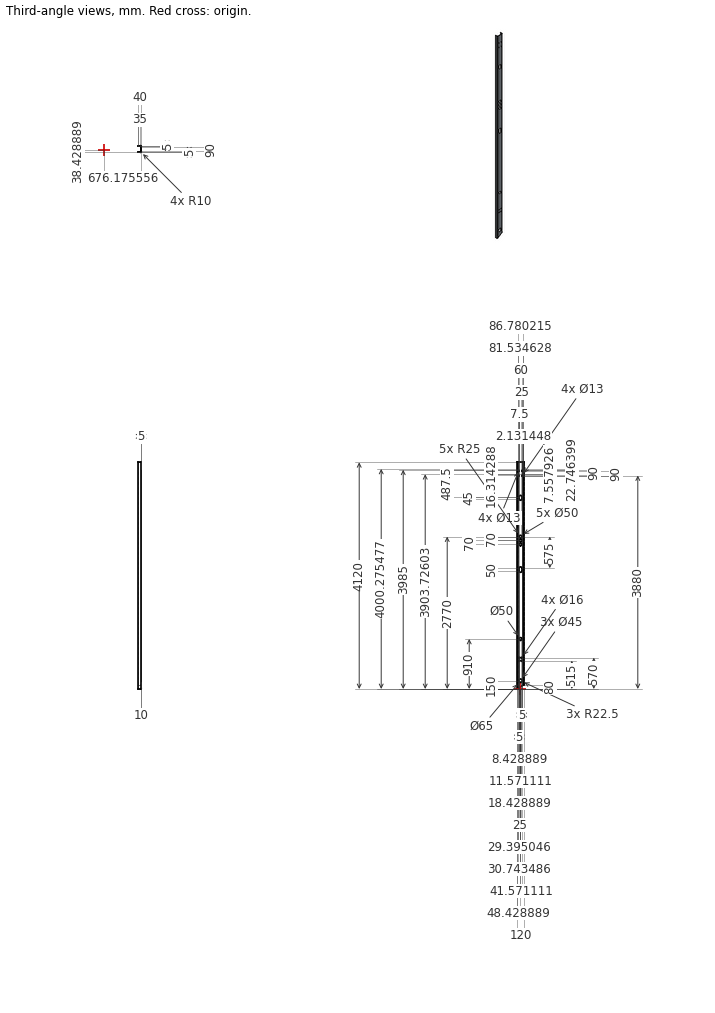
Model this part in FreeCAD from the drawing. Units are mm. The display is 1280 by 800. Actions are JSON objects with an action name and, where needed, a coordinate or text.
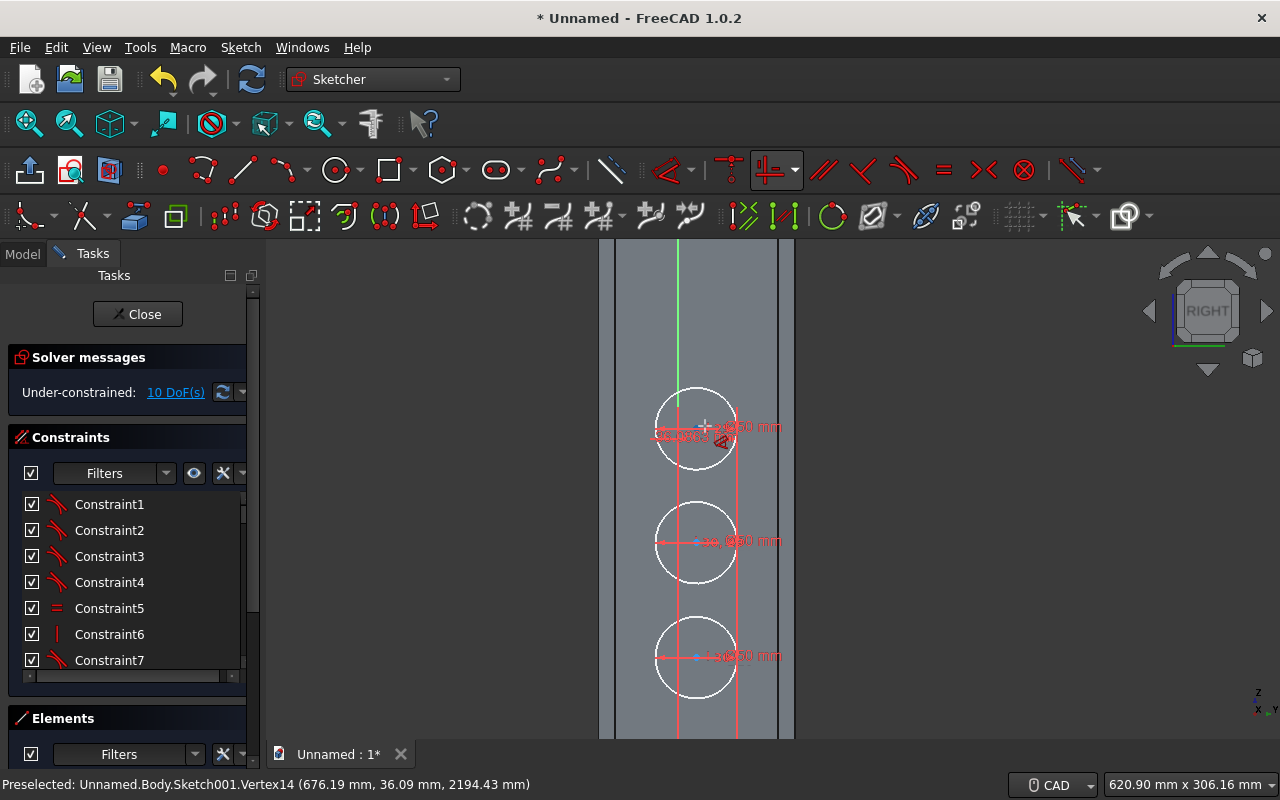
{"action": "left_click", "coordinate": [696, 429]}
{"action": "left_click", "coordinate": [716, 371]}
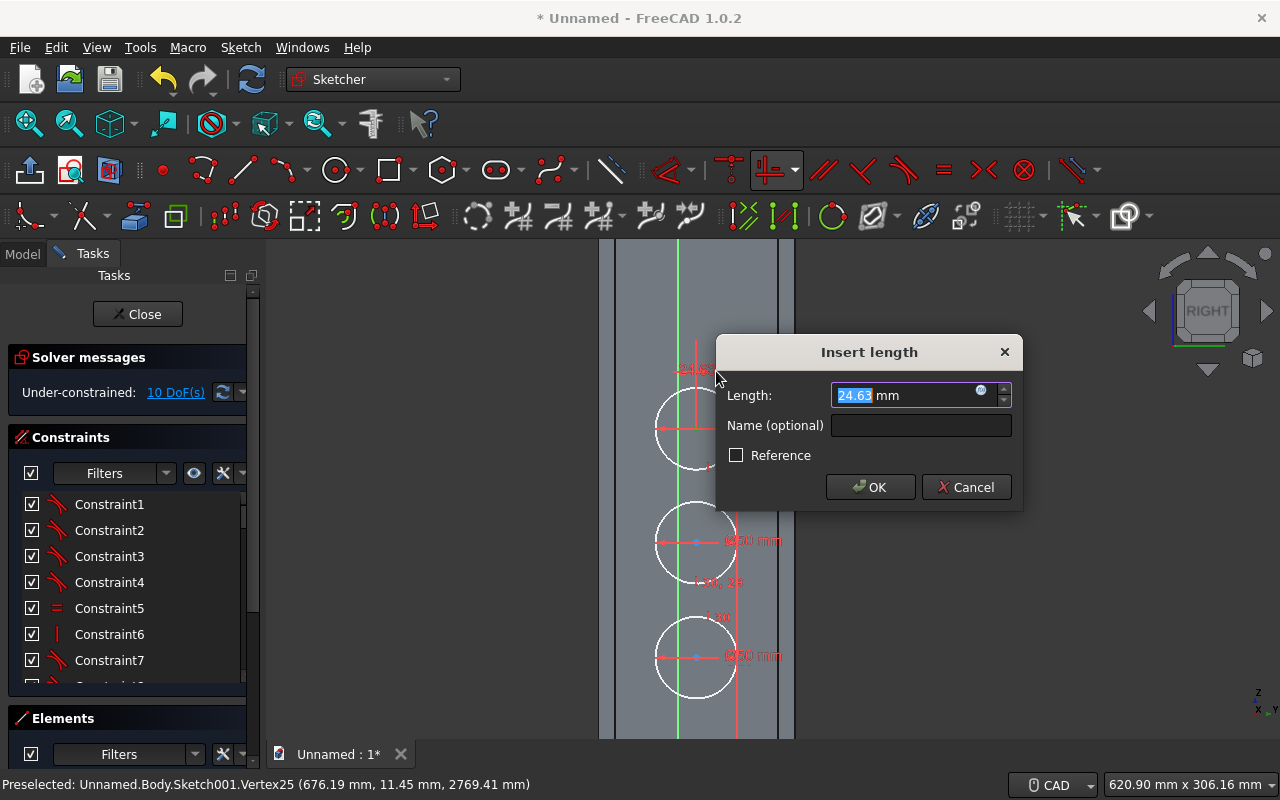
{"action": "type", "text": "25"}
{"action": "key", "text": "Return"}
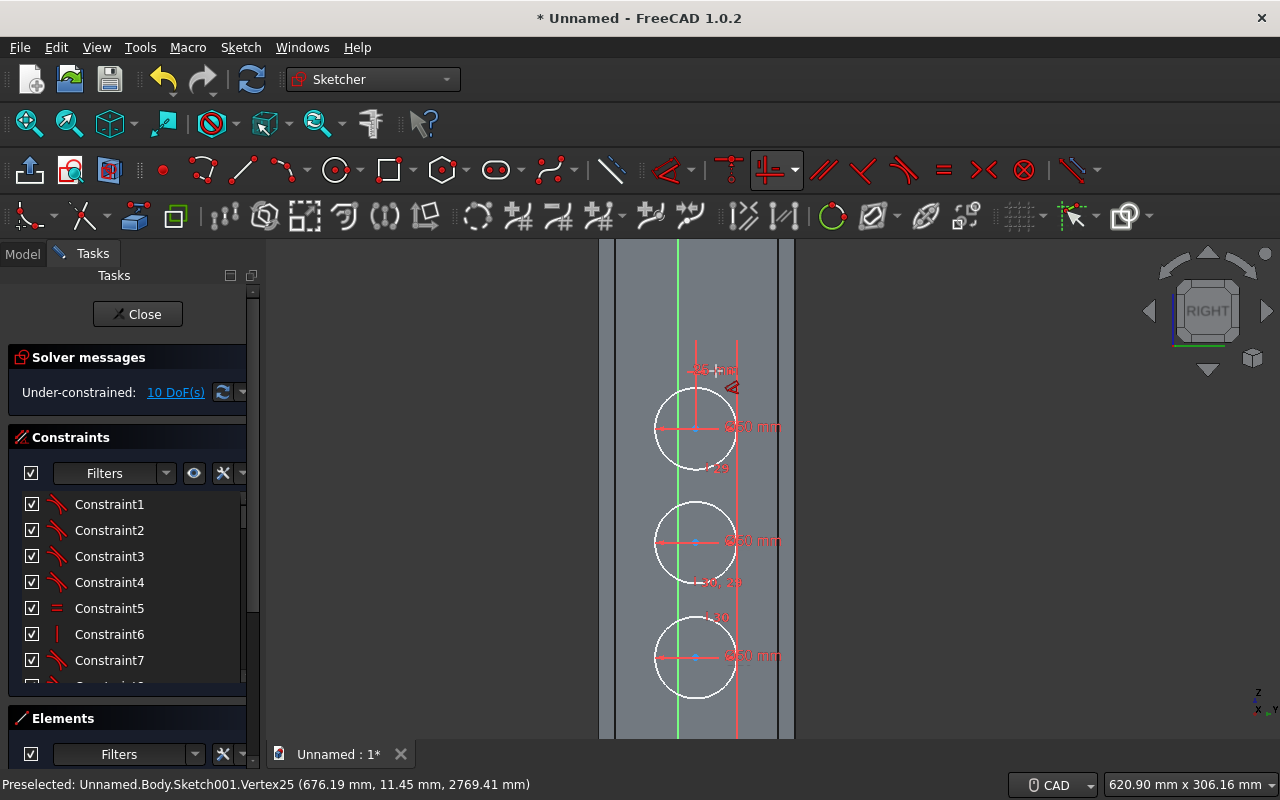
{"action": "scroll", "coordinate": [705, 426], "scroll_direction": "down", "scroll_amount": 15}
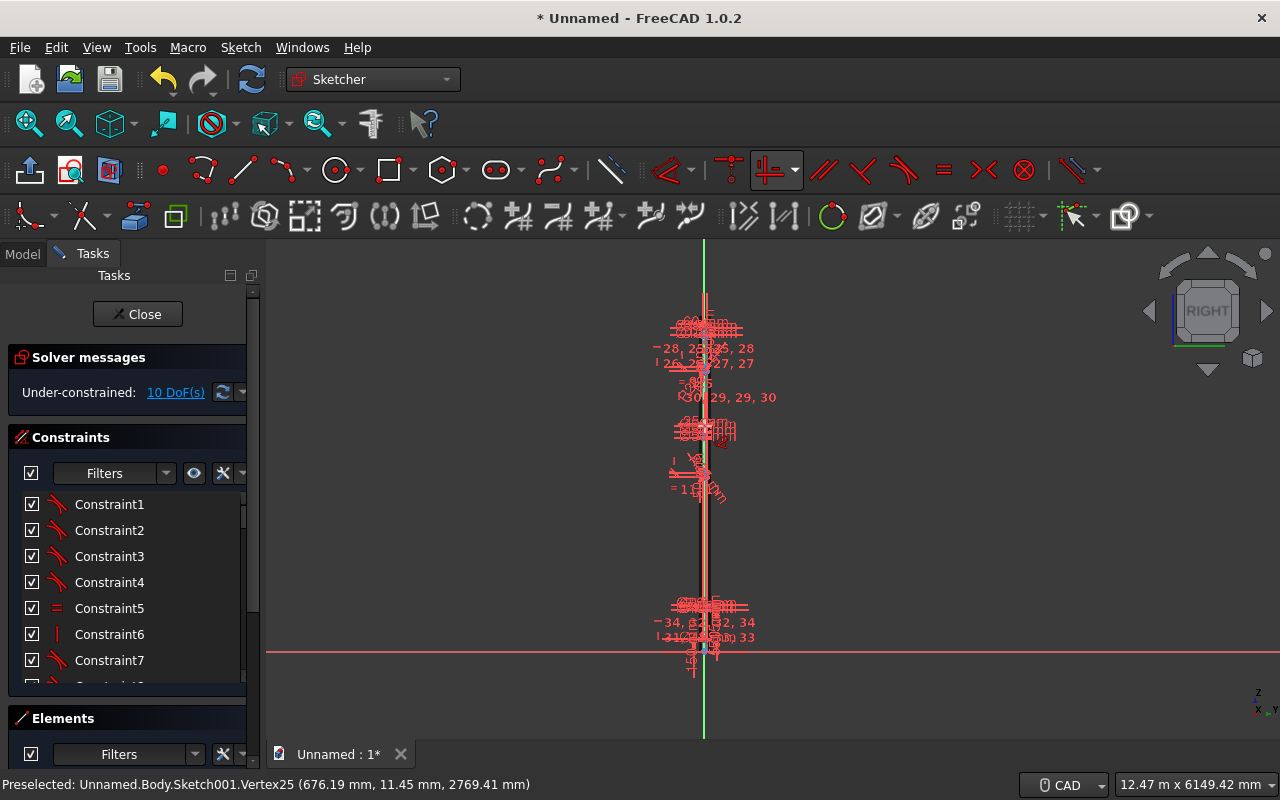
{"action": "scroll", "coordinate": [705, 426], "scroll_direction": "up", "scroll_amount": 10}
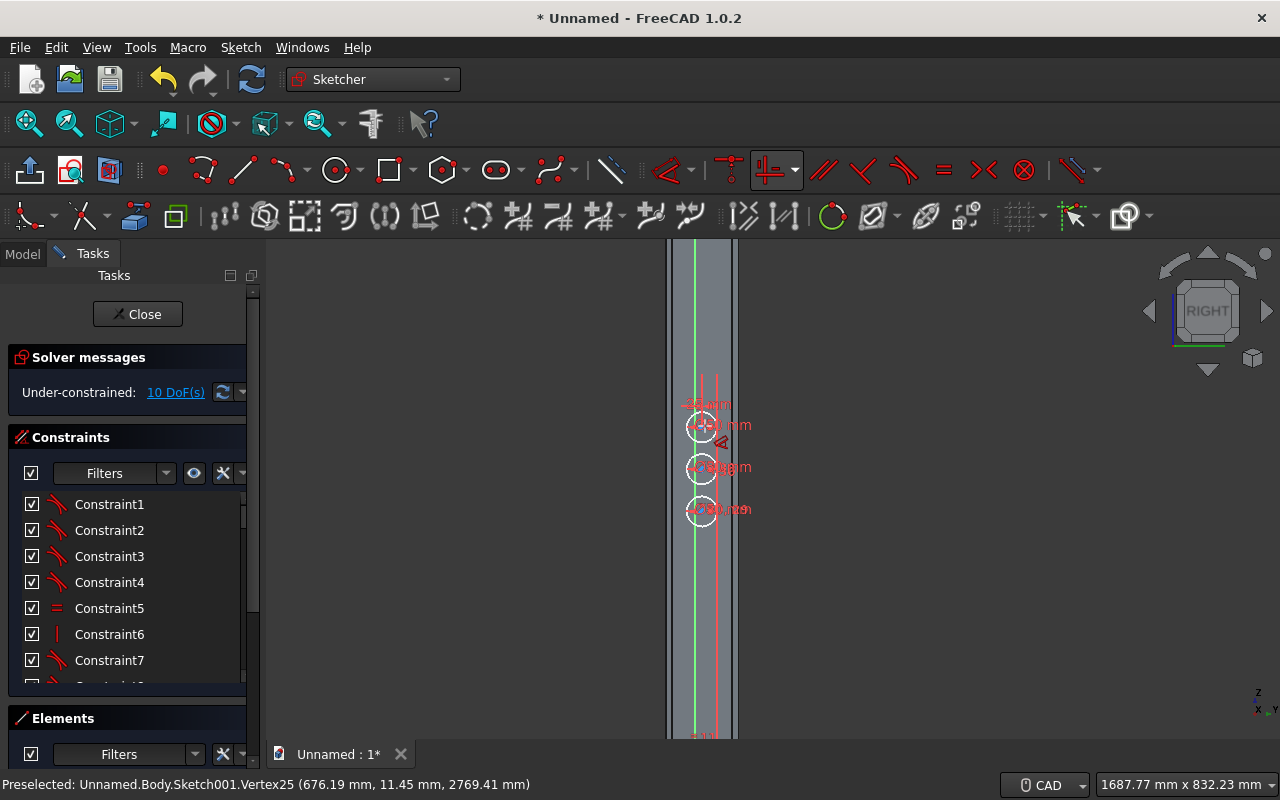
{"action": "left_click", "coordinate": [702, 427]}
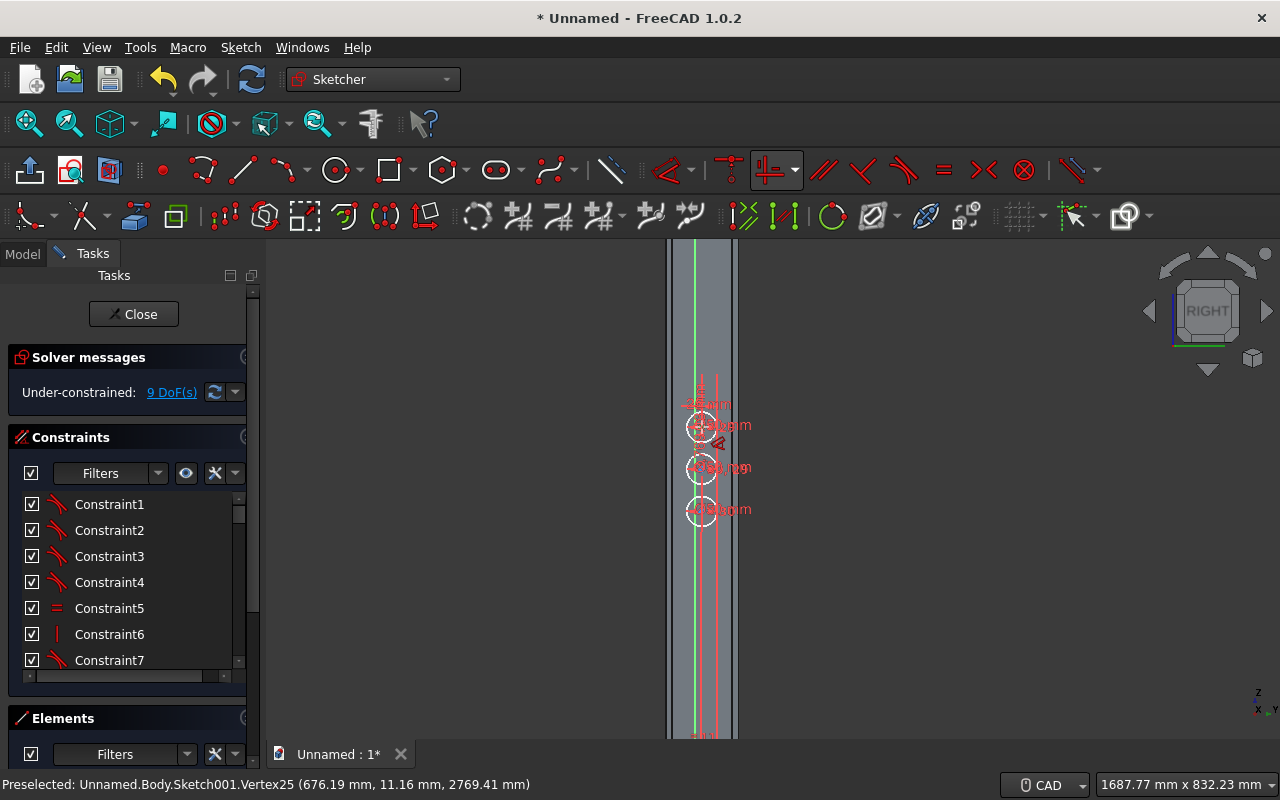
{"action": "left_click", "coordinate": [702, 469]}
{"action": "left_click", "coordinate": [668, 448]}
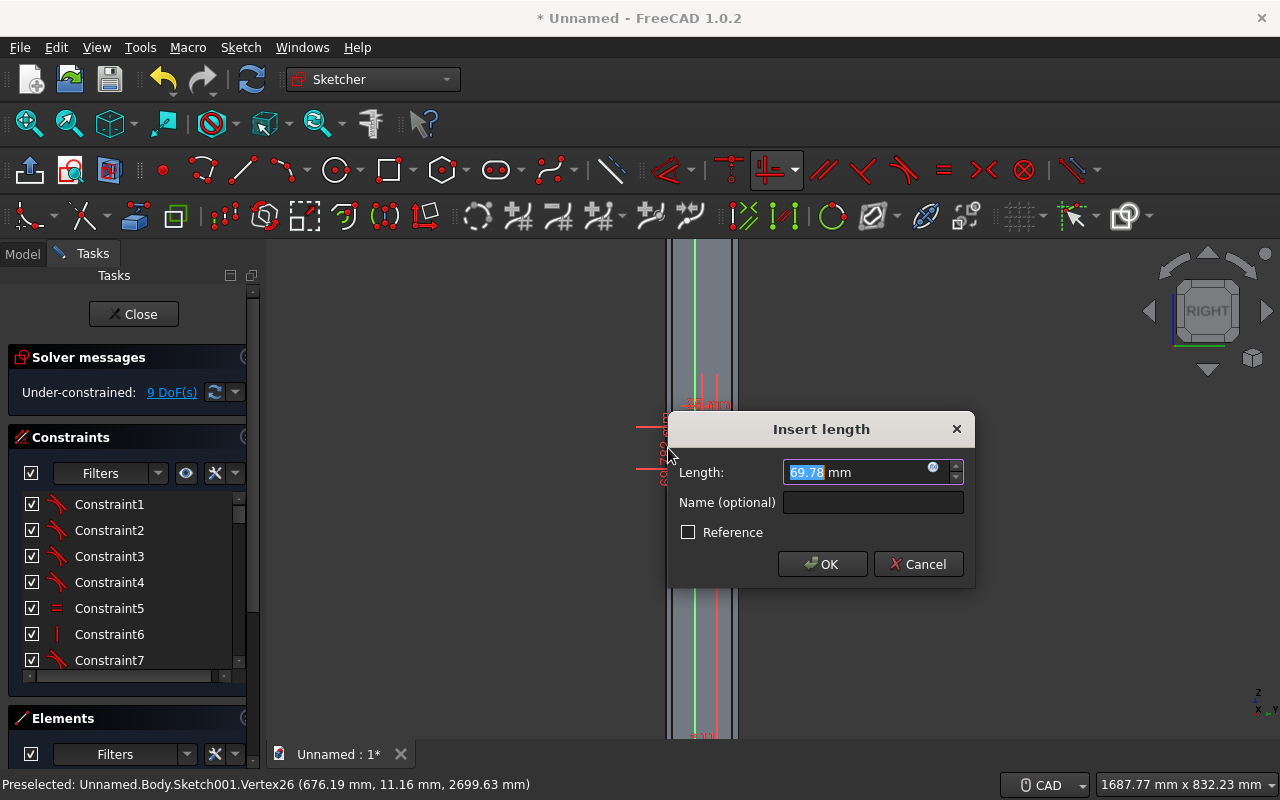
{"action": "type", "text": "70"}
{"action": "key", "text": "Return"}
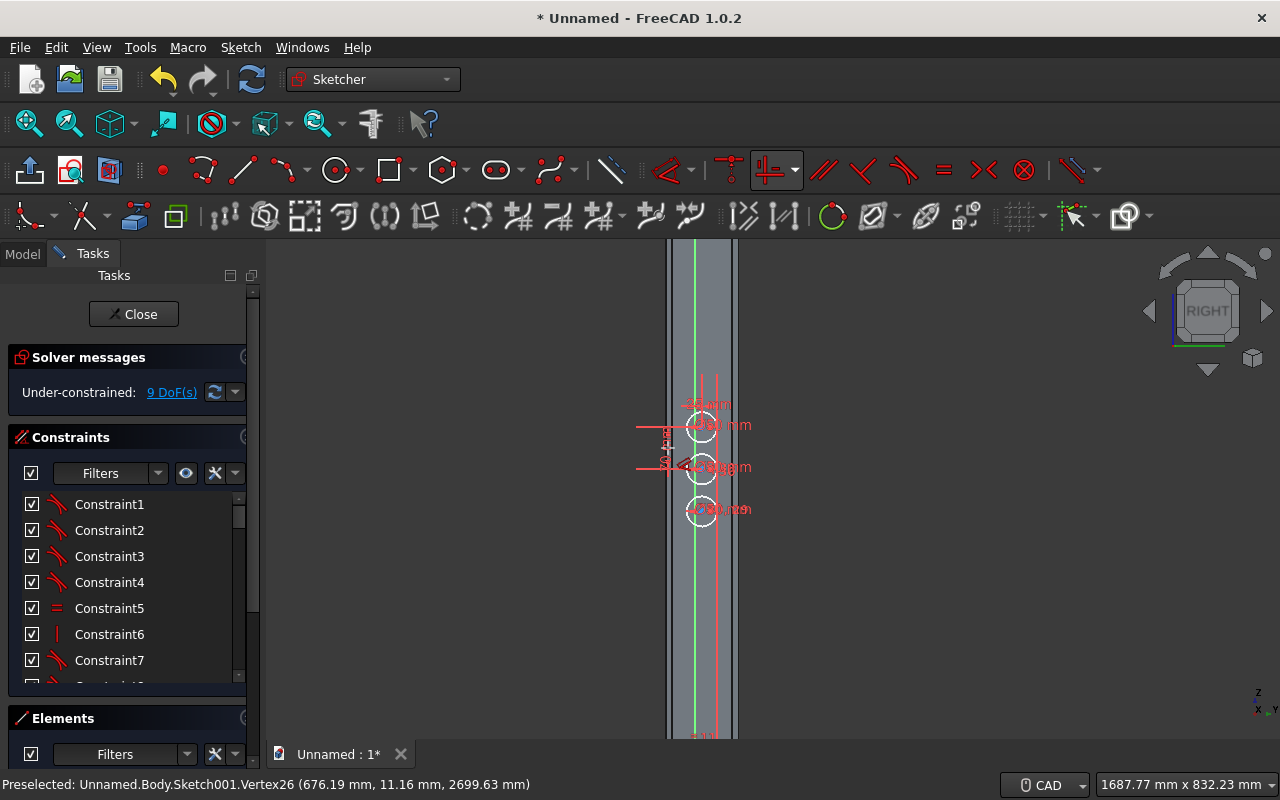
{"action": "left_click", "coordinate": [702, 469]}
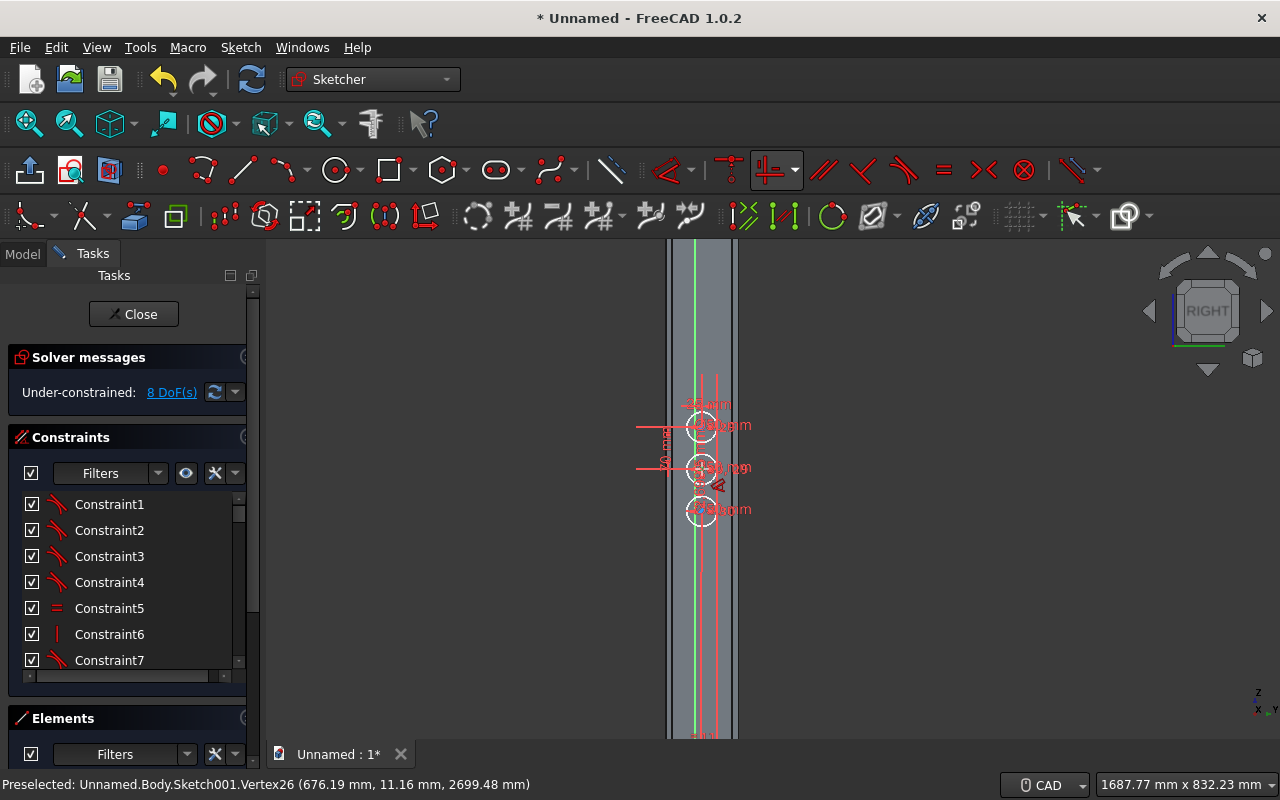
{"action": "left_click", "coordinate": [702, 511]}
{"action": "left_click", "coordinate": [668, 490]}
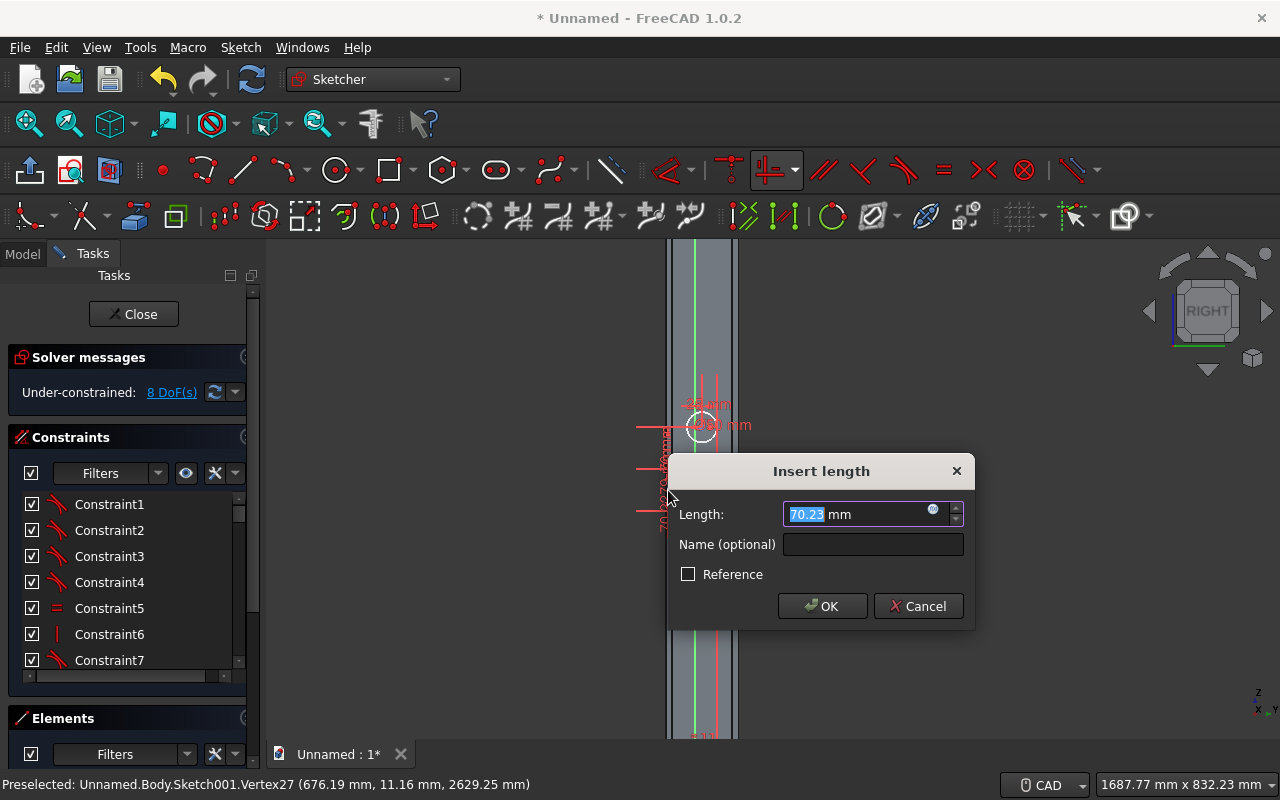
{"action": "type", "text": "70"}
{"action": "key", "text": "Return"}